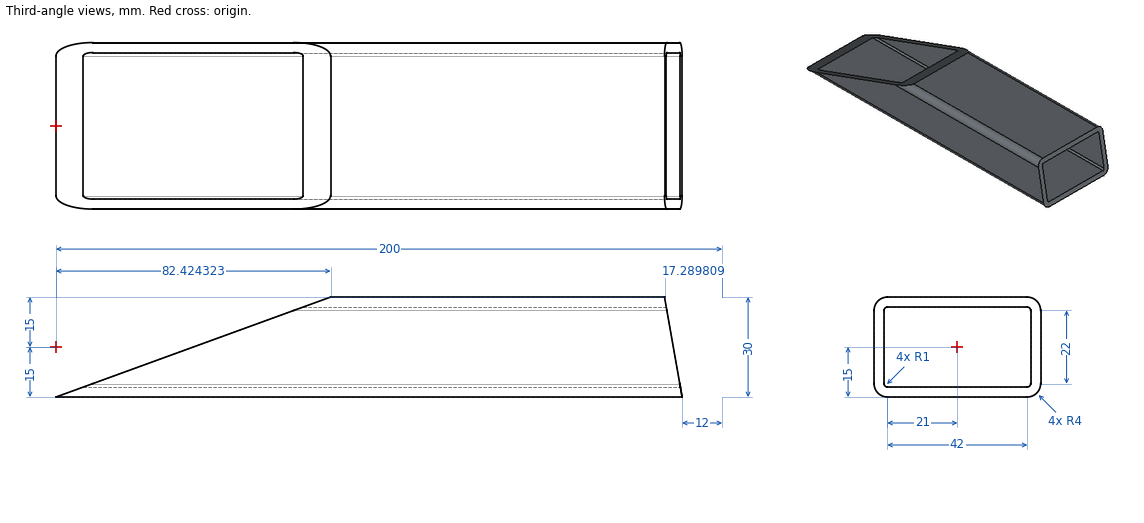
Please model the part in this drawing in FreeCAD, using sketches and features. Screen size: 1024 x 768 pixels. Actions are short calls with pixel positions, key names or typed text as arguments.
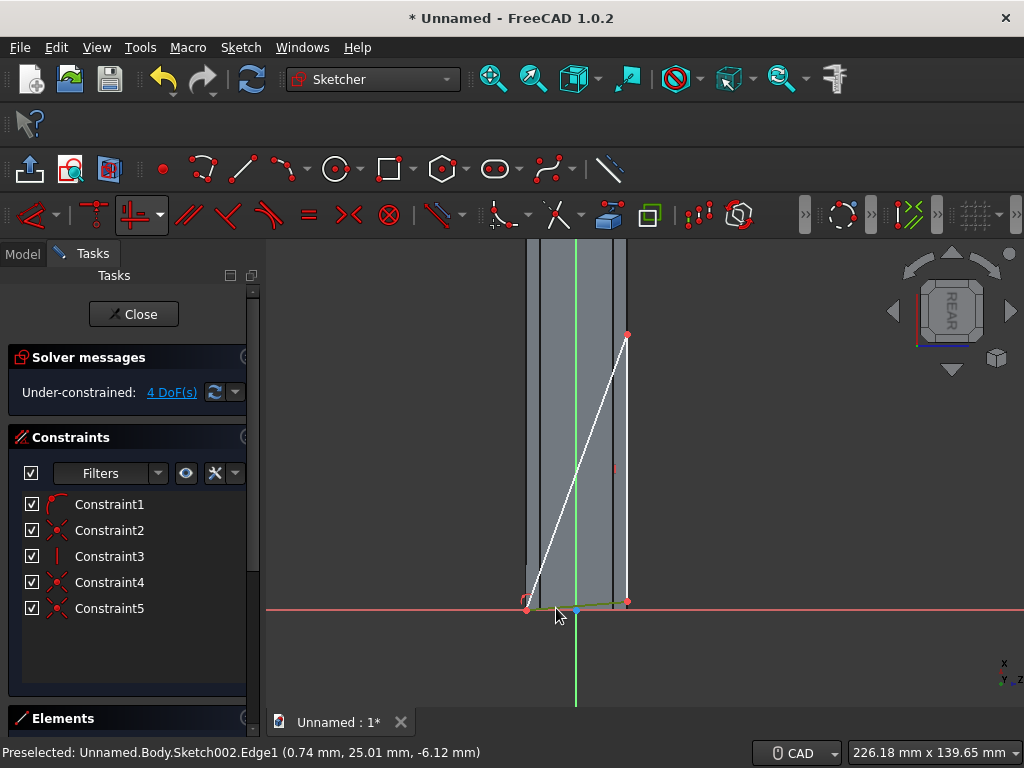
click(162, 216)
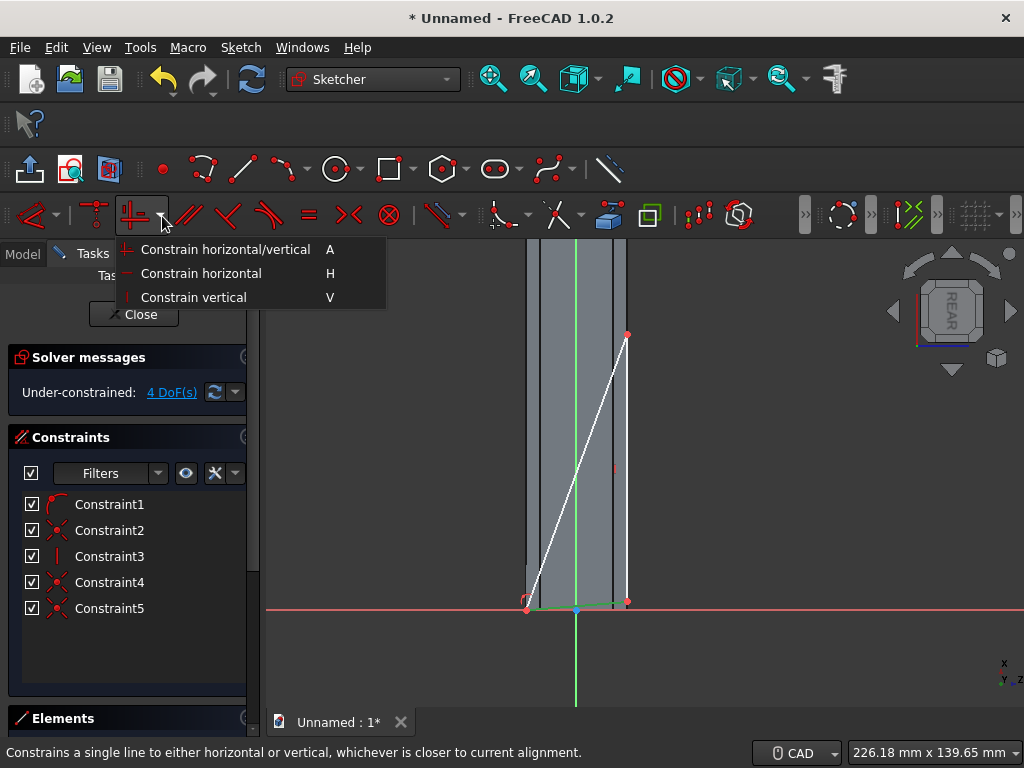
click(251, 273)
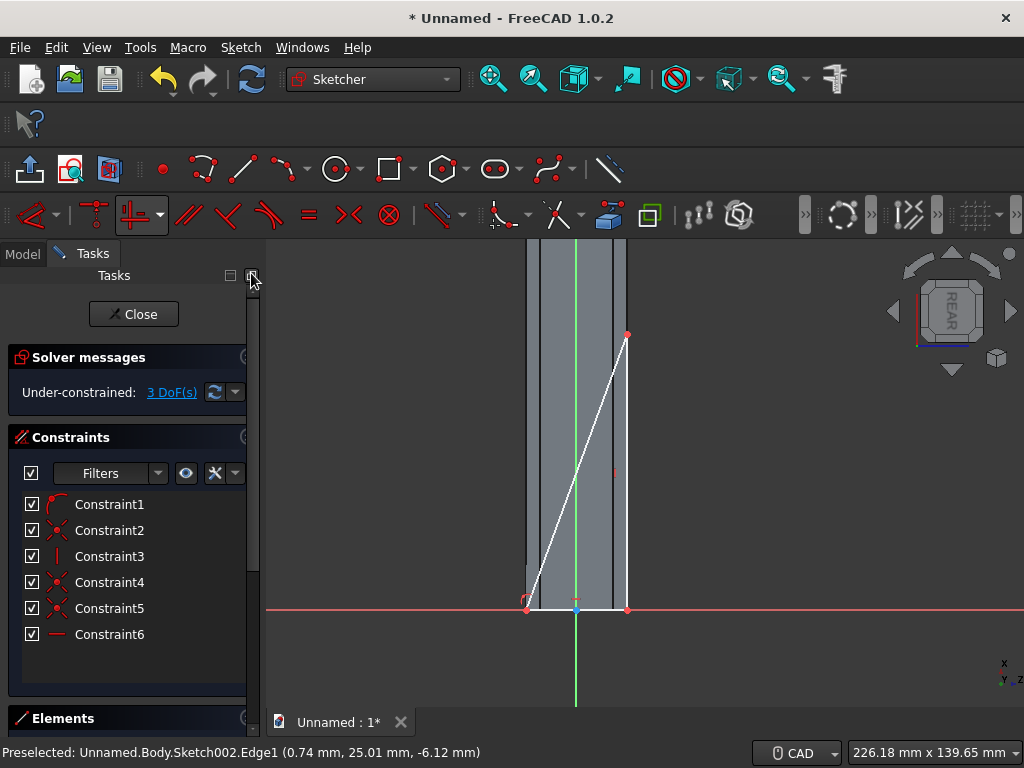
click(32, 216)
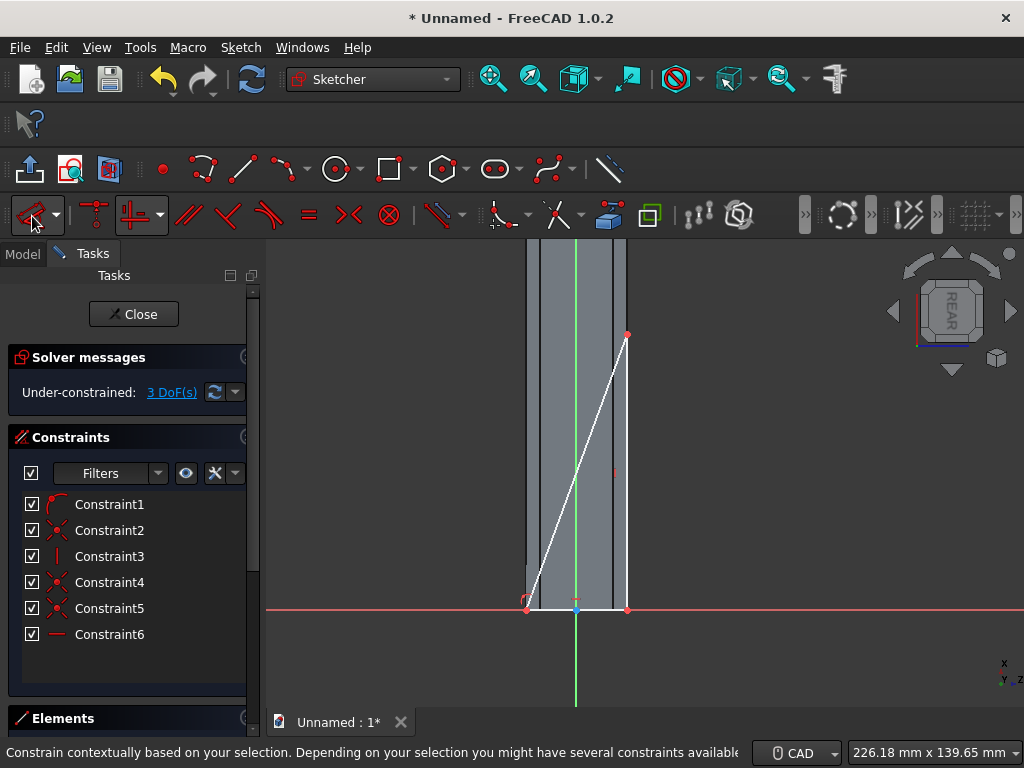
click(556, 610)
click(553, 644)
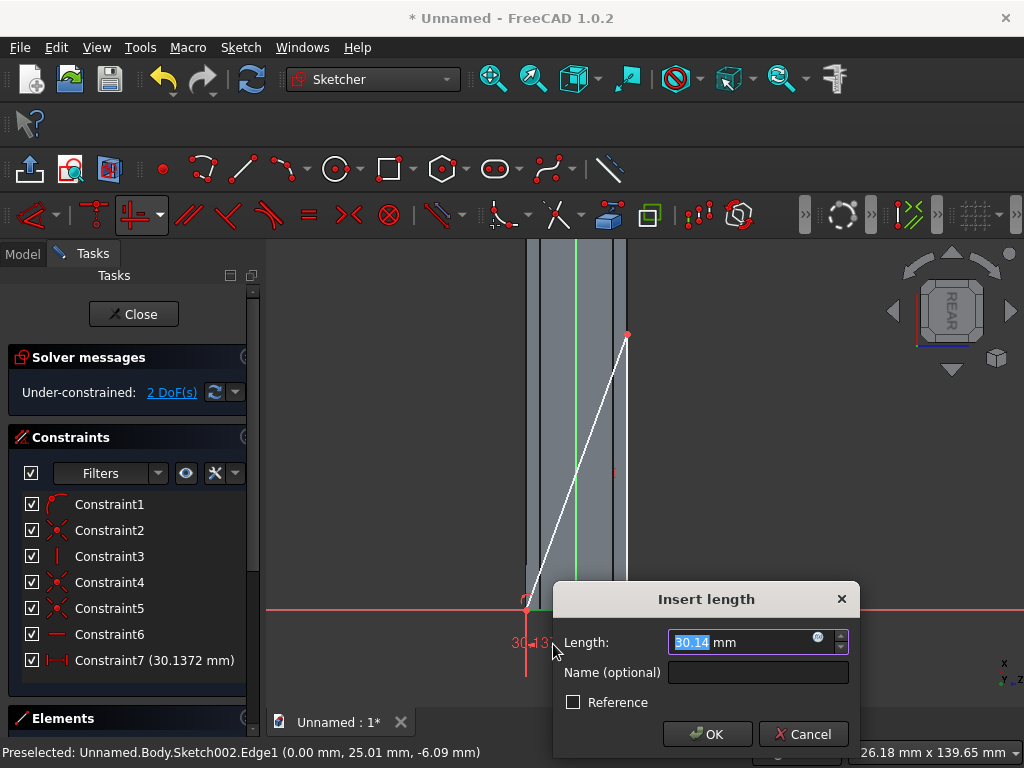
text(30)
key(Return)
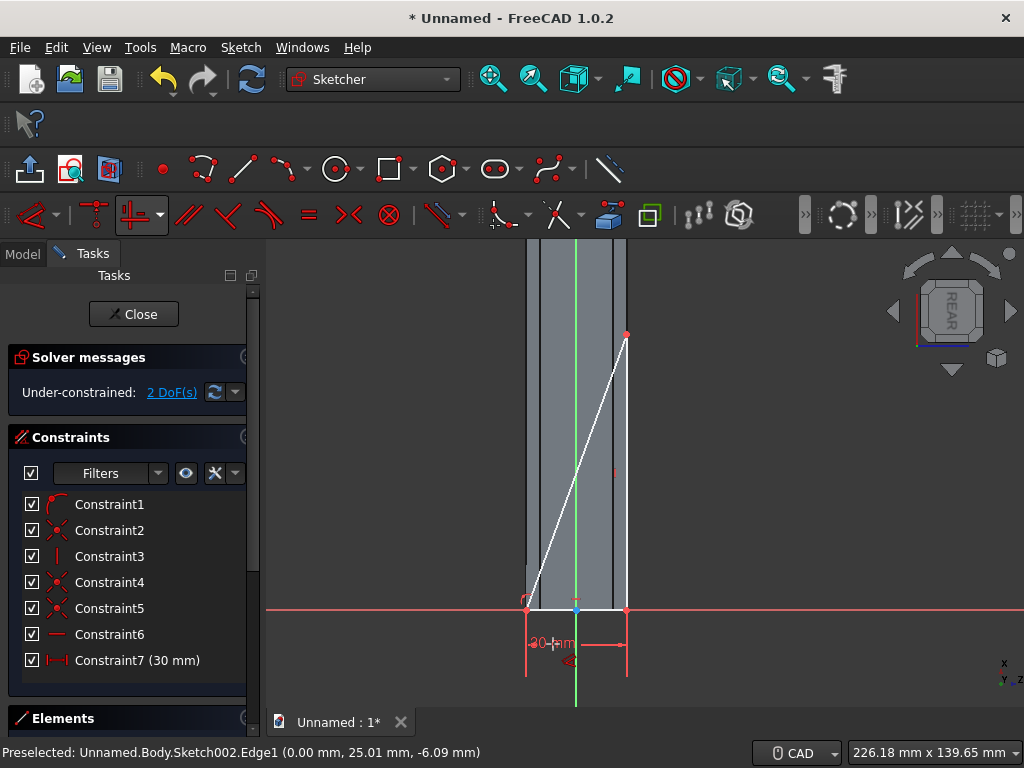
click(526, 610)
click(563, 576)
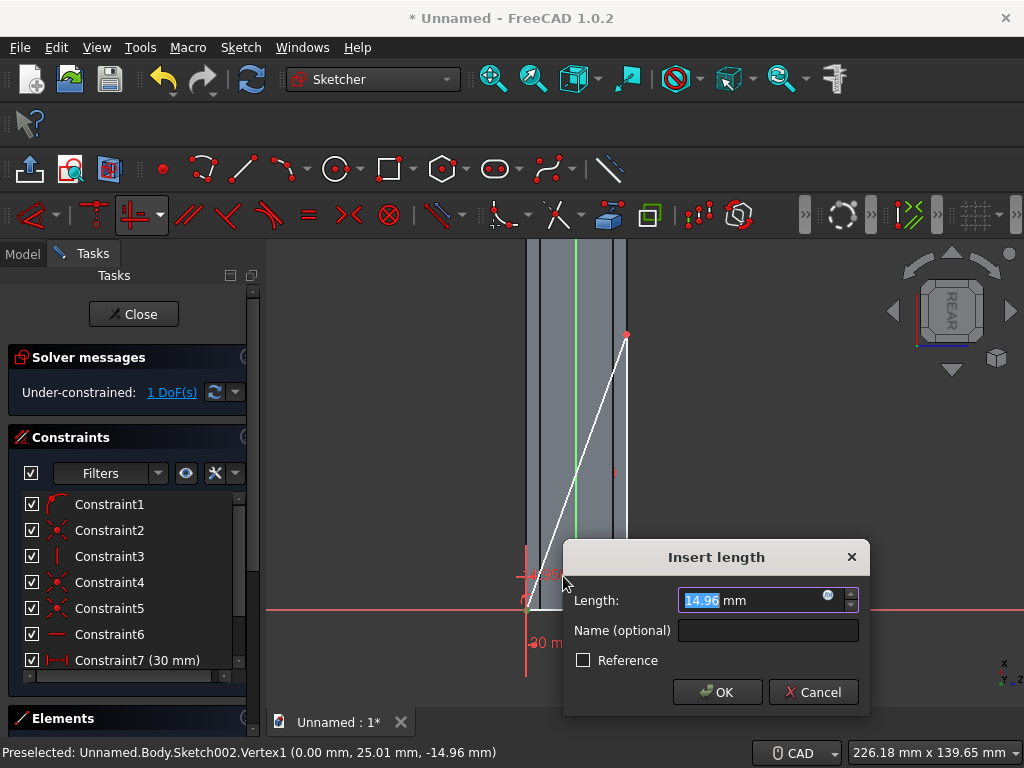
text(15)
key(Return)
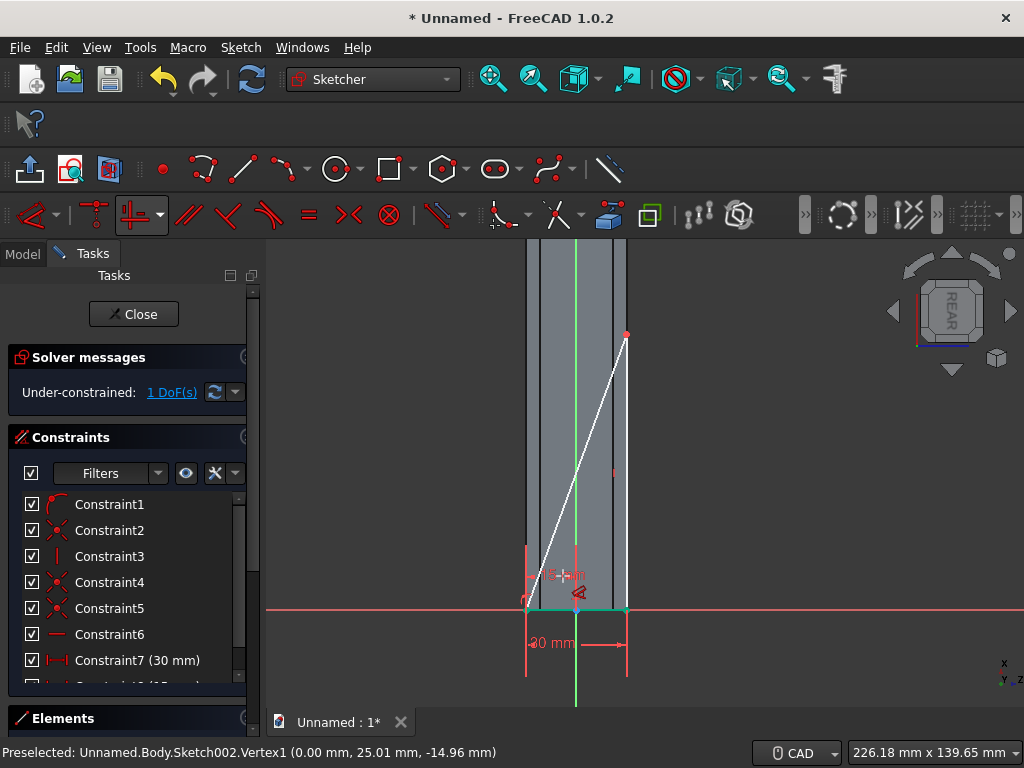
click(627, 528)
click(661, 473)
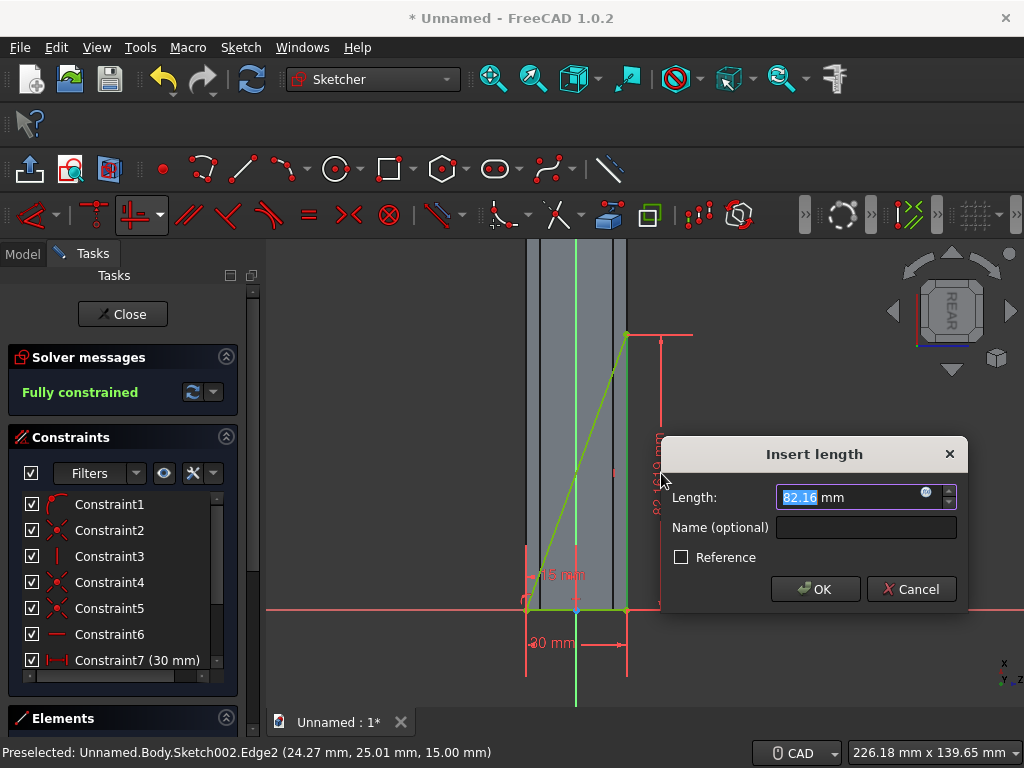
text(82.424323)
key(Return)
key(Escape)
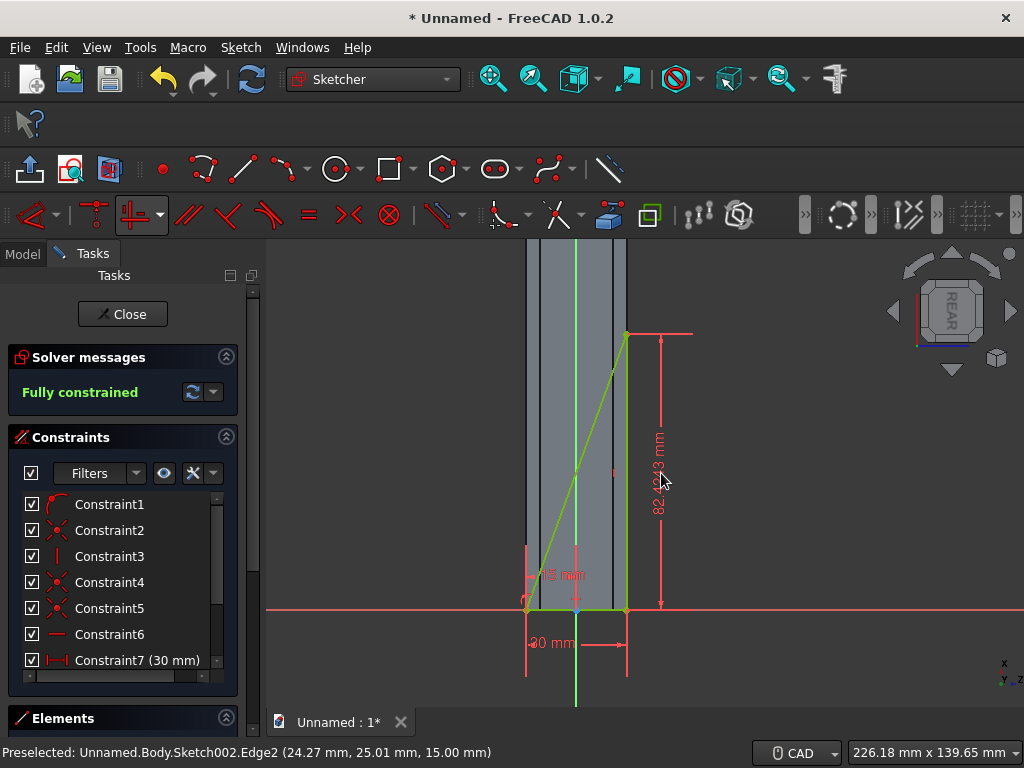
click(123, 314)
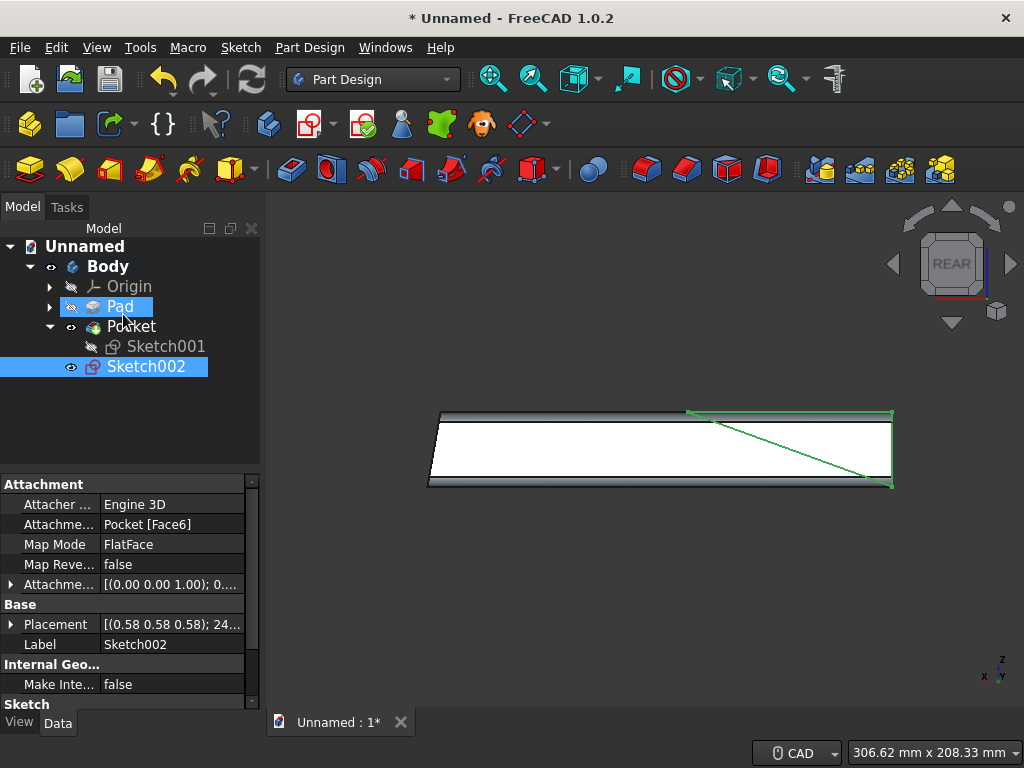
click(292, 170)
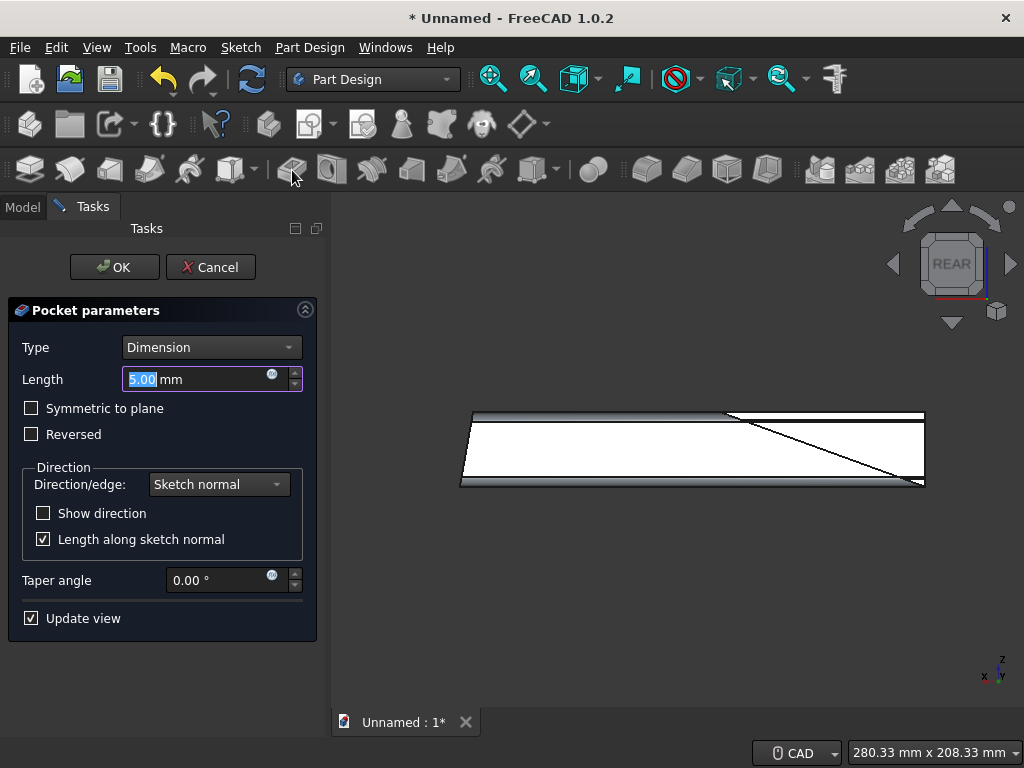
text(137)
key(Tab)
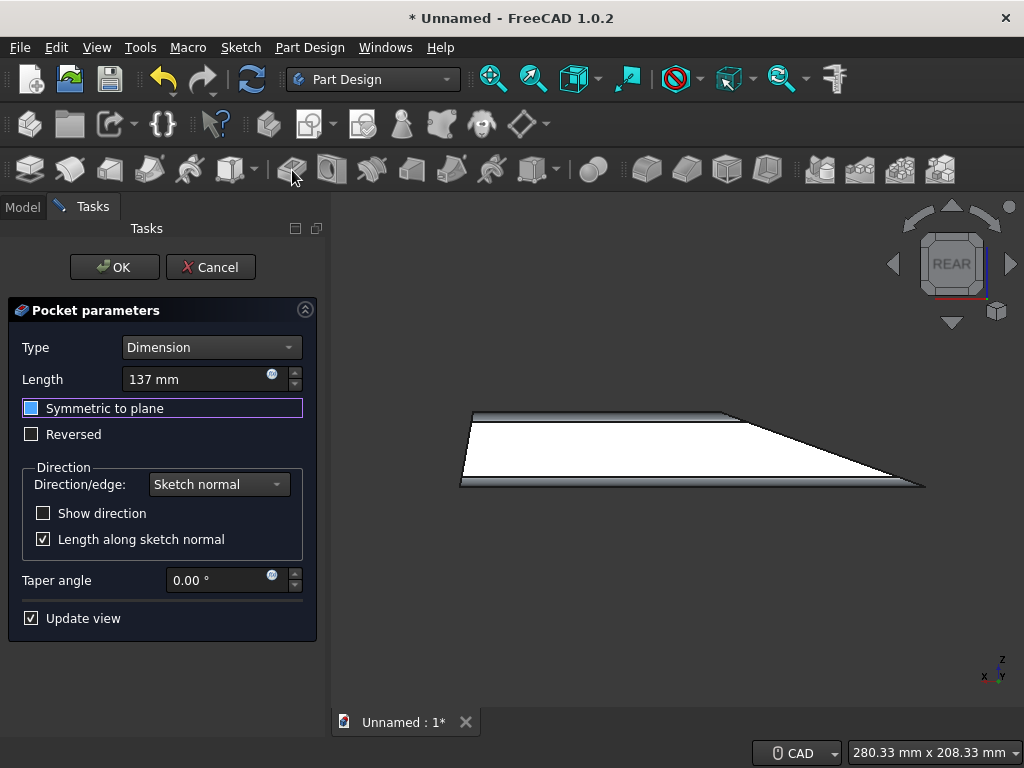
click(115, 267)